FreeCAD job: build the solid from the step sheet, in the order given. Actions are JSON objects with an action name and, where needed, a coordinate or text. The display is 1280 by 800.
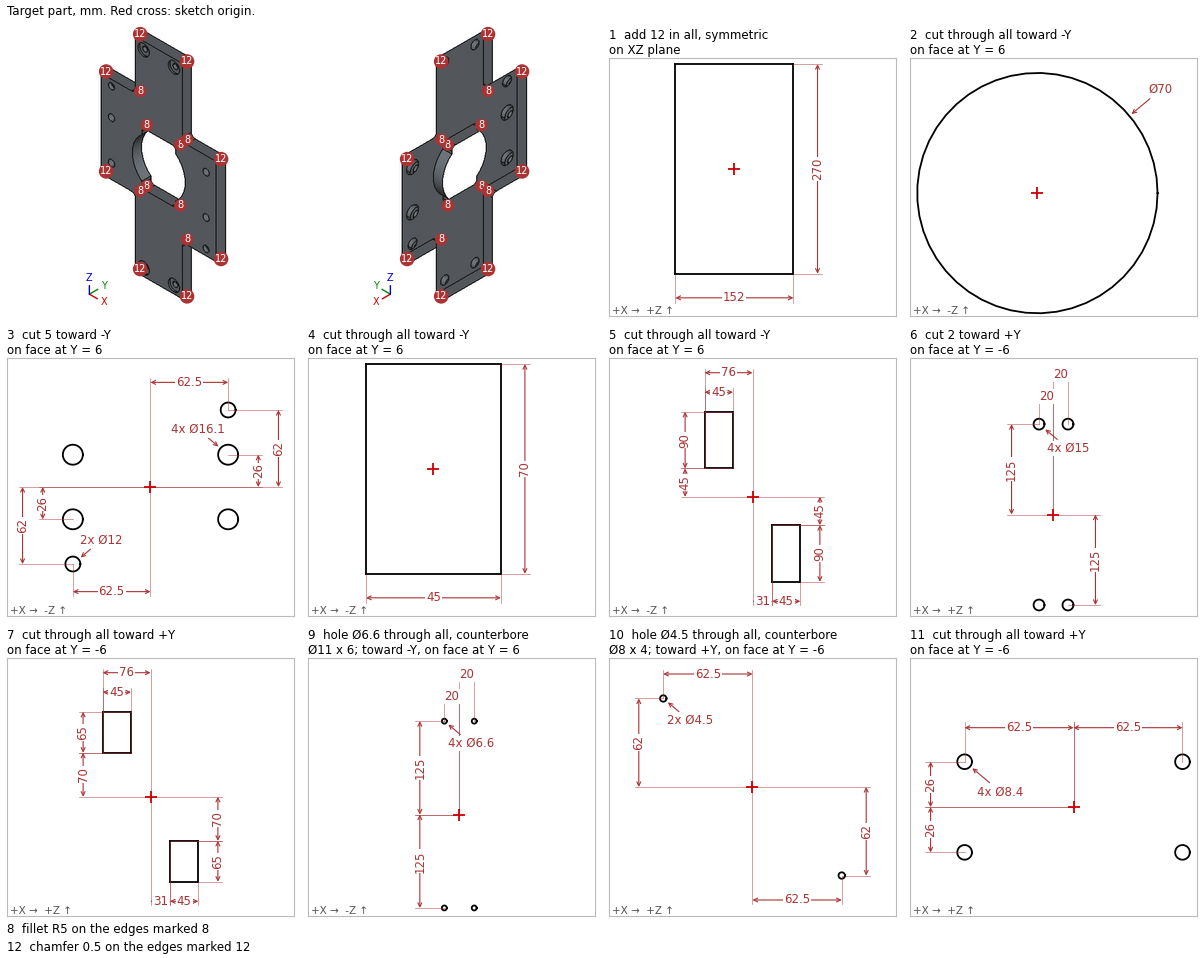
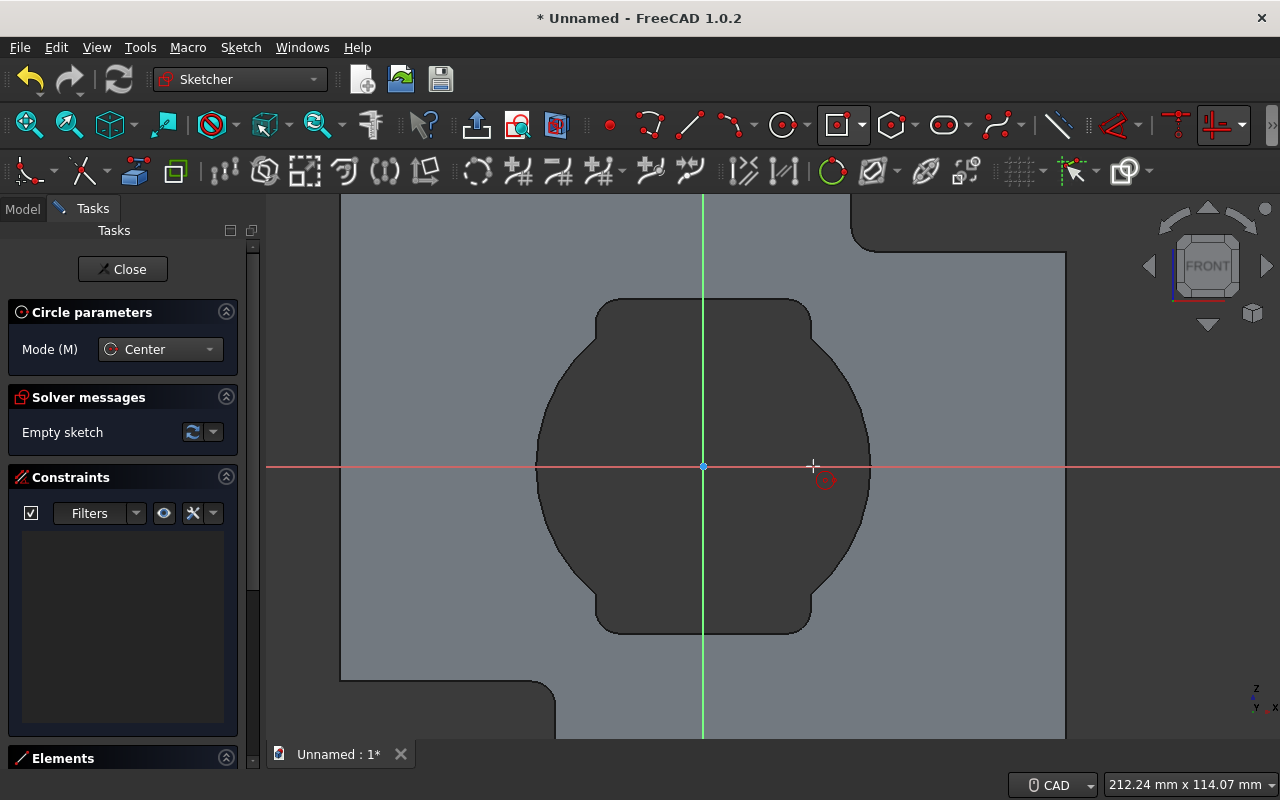
{"action": "left_click", "coordinate": [405, 342]}
{"action": "mouse_move", "coordinate": [419, 328]}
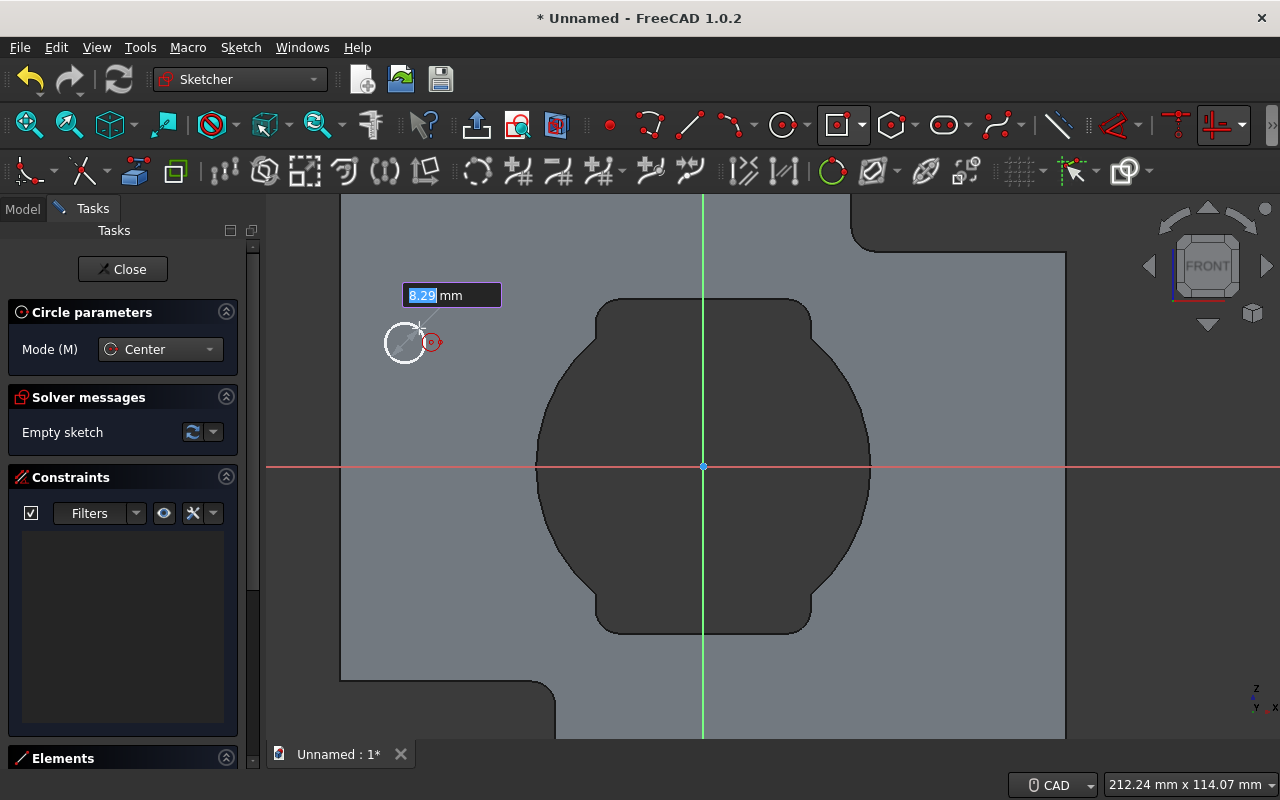
{"action": "type", "text": "8.4"}
{"action": "key", "text": "Return"}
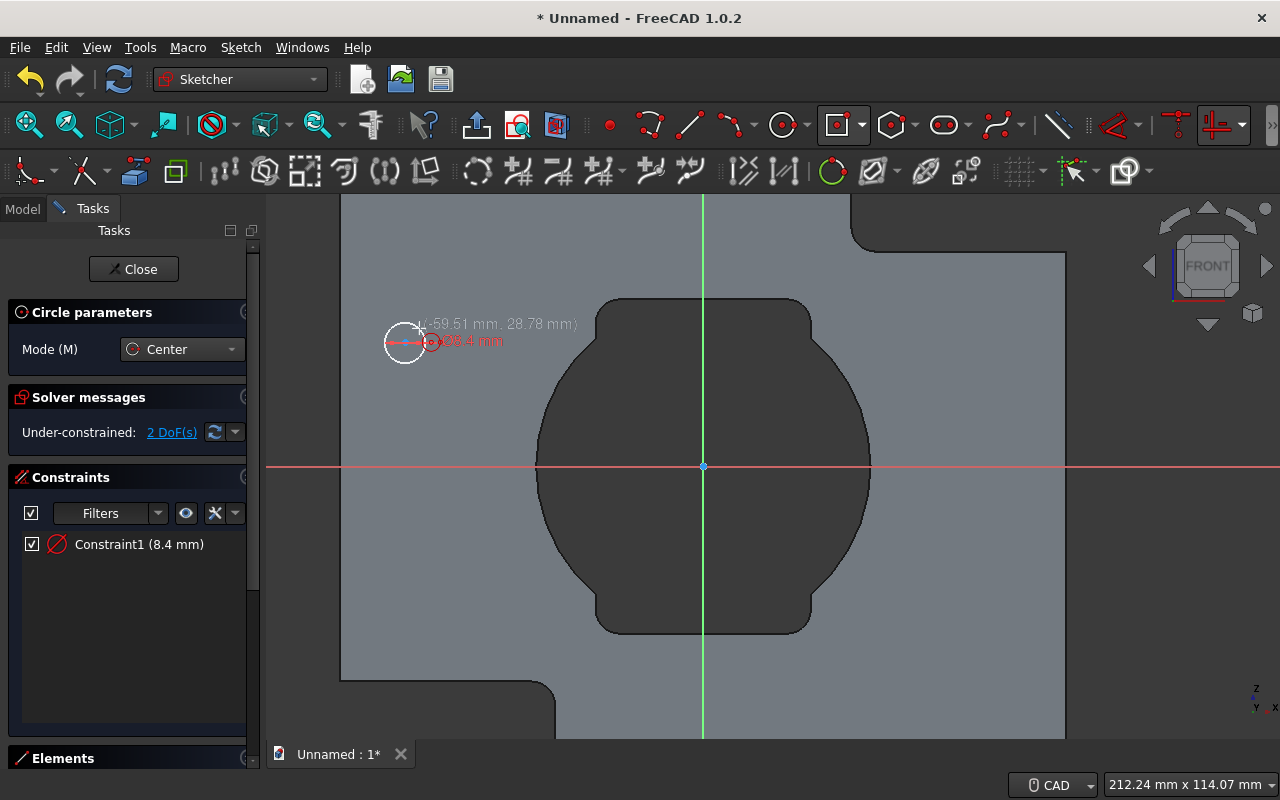
{"action": "left_click", "coordinate": [405, 591]}
{"action": "mouse_move", "coordinate": [419, 577]}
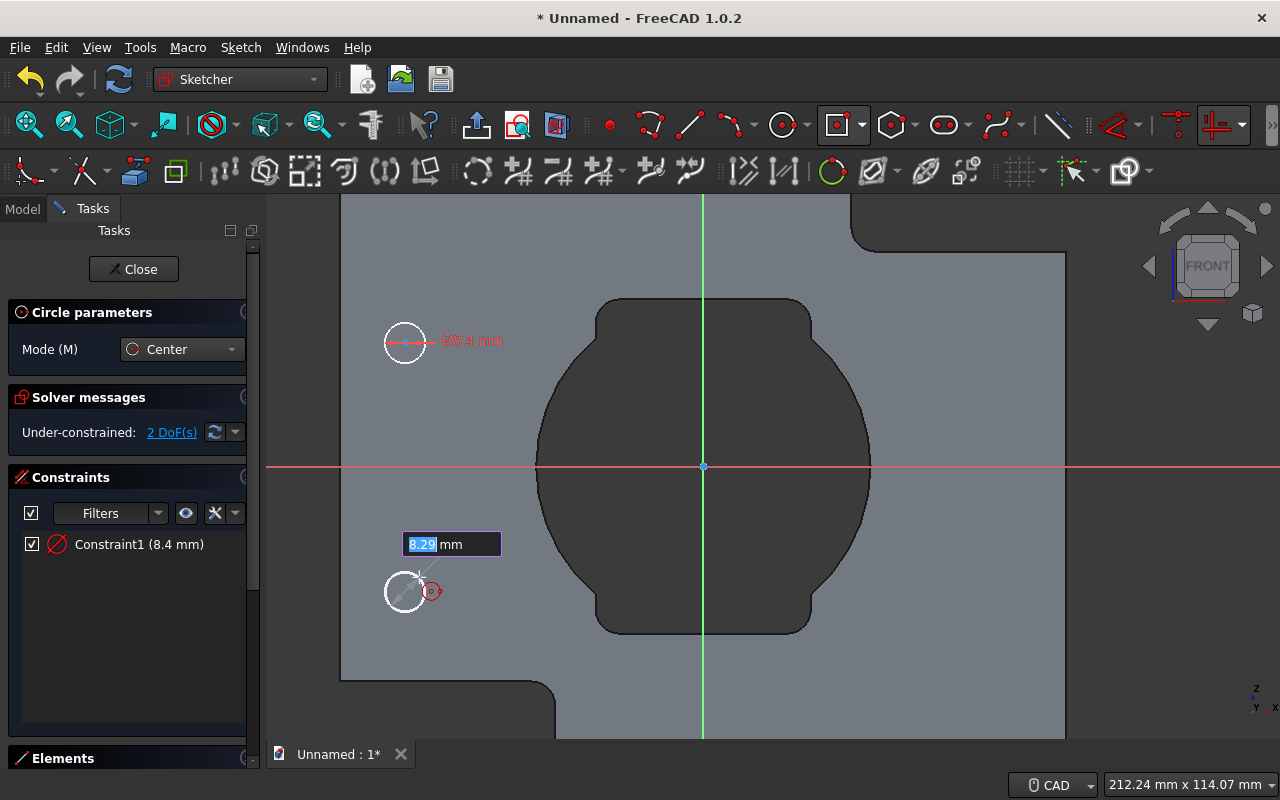
{"action": "type", "text": "8.4"}
{"action": "key", "text": "Return"}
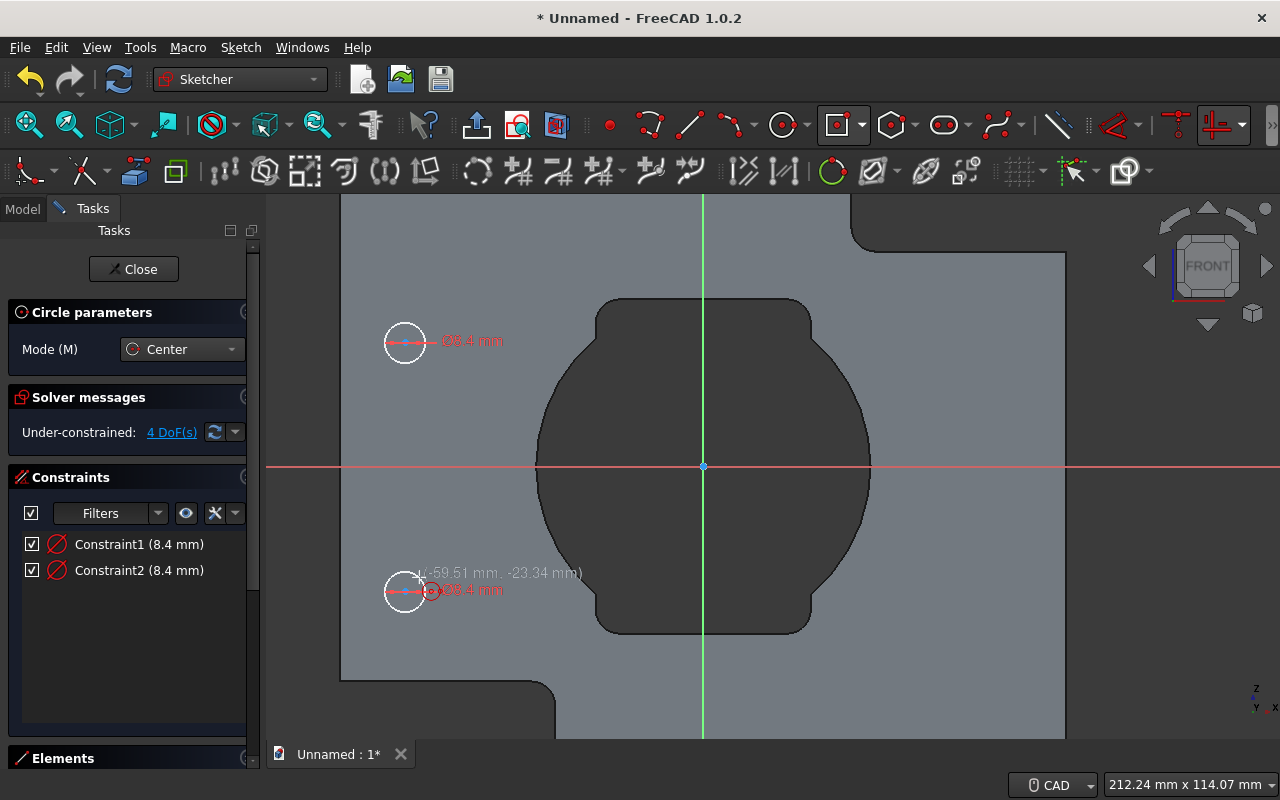
{"action": "left_click", "coordinate": [1002, 342]}
{"action": "mouse_move", "coordinate": [1016, 328]}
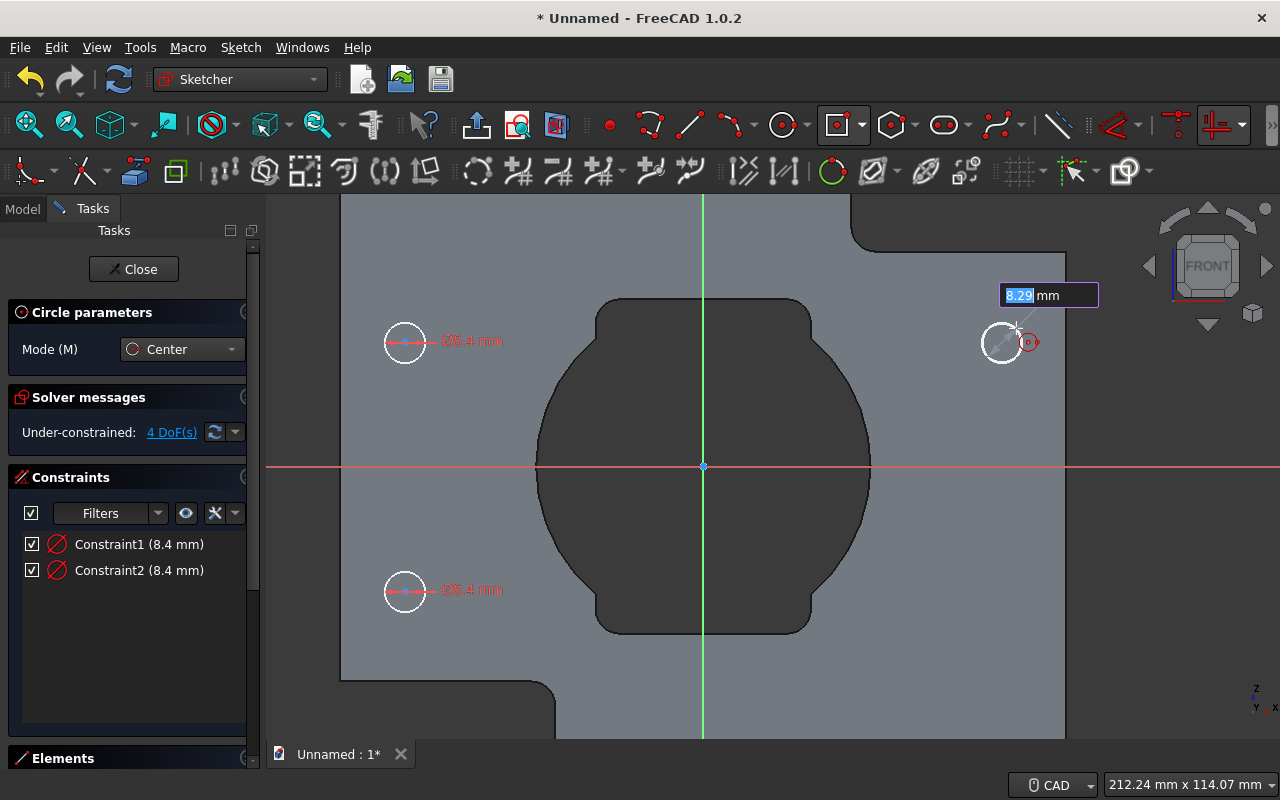
{"action": "type", "text": "8.4"}
{"action": "key", "text": "Return"}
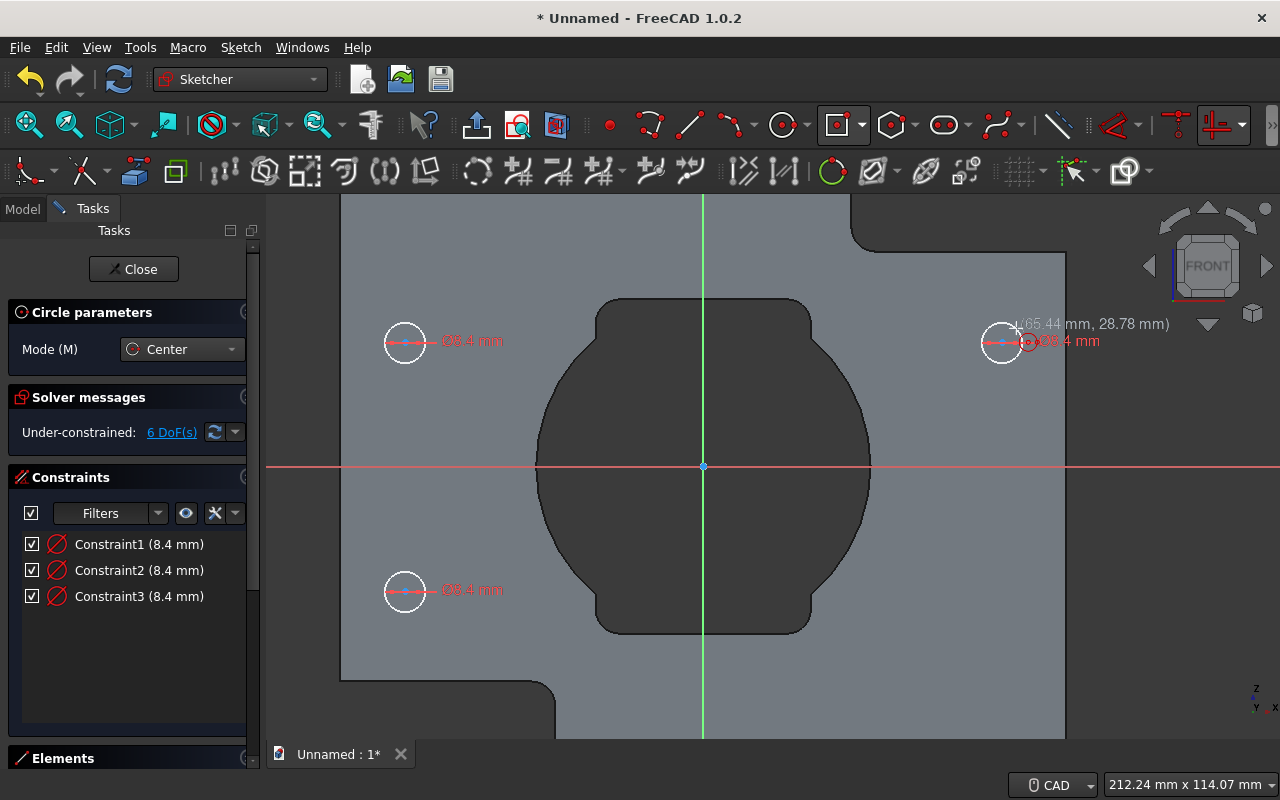
{"action": "left_click", "coordinate": [1002, 591]}
{"action": "mouse_move", "coordinate": [1016, 577]}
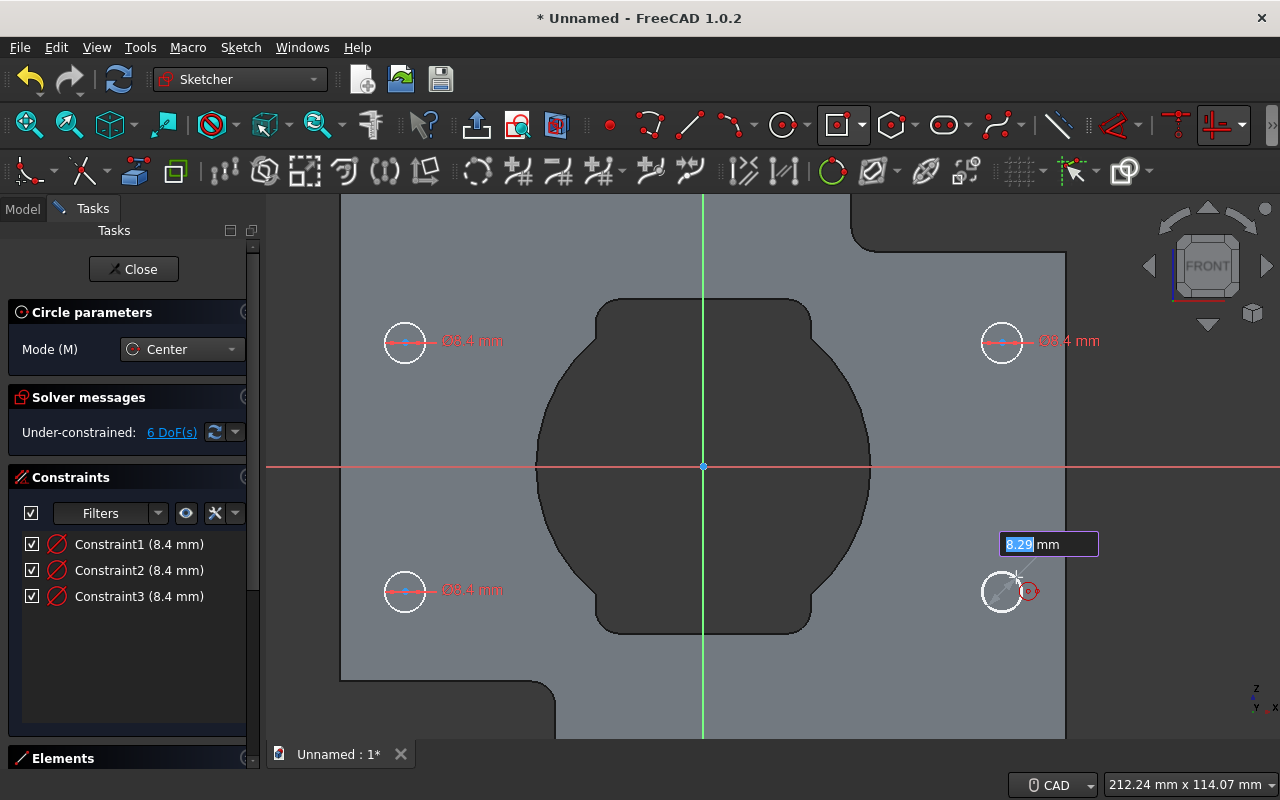
{"action": "type", "text": "8.4"}
{"action": "key", "text": "Return"}
{"action": "key", "text": "Escape"}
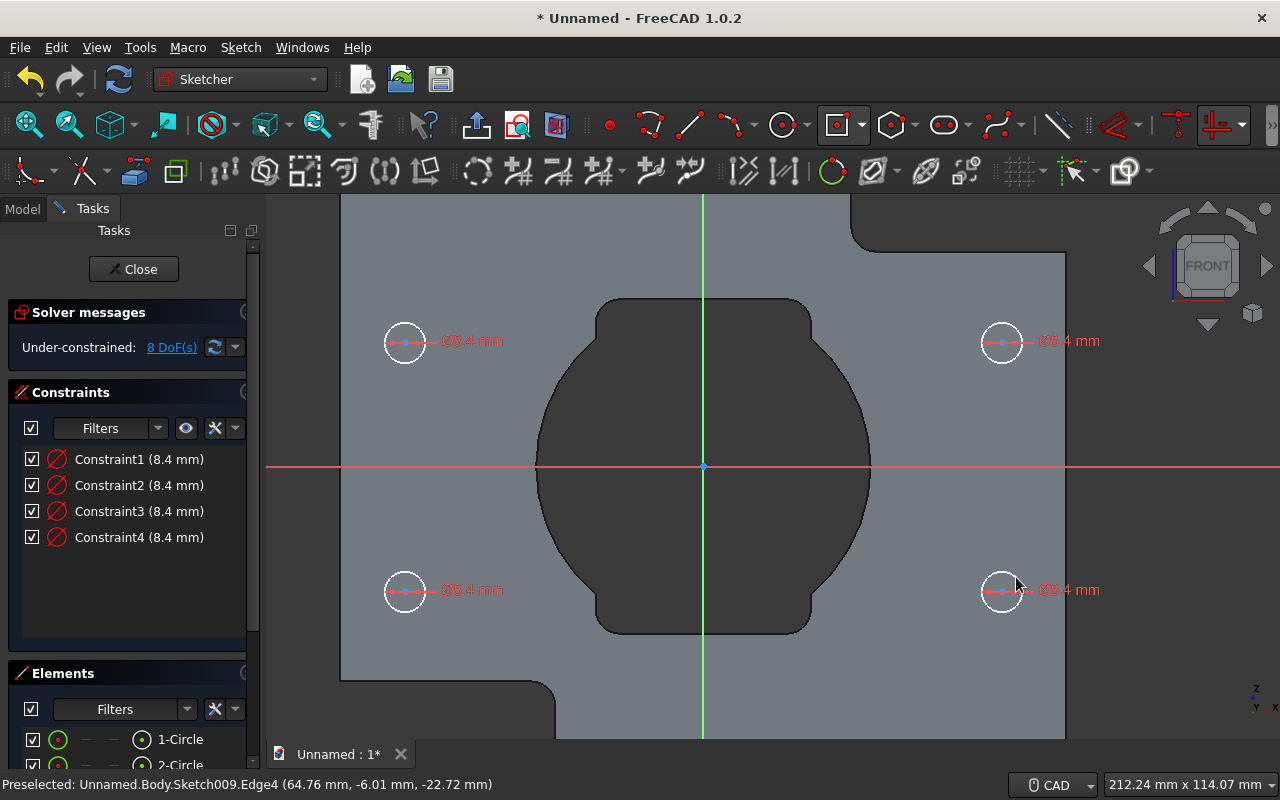
{"action": "left_click", "coordinate": [405, 343]}